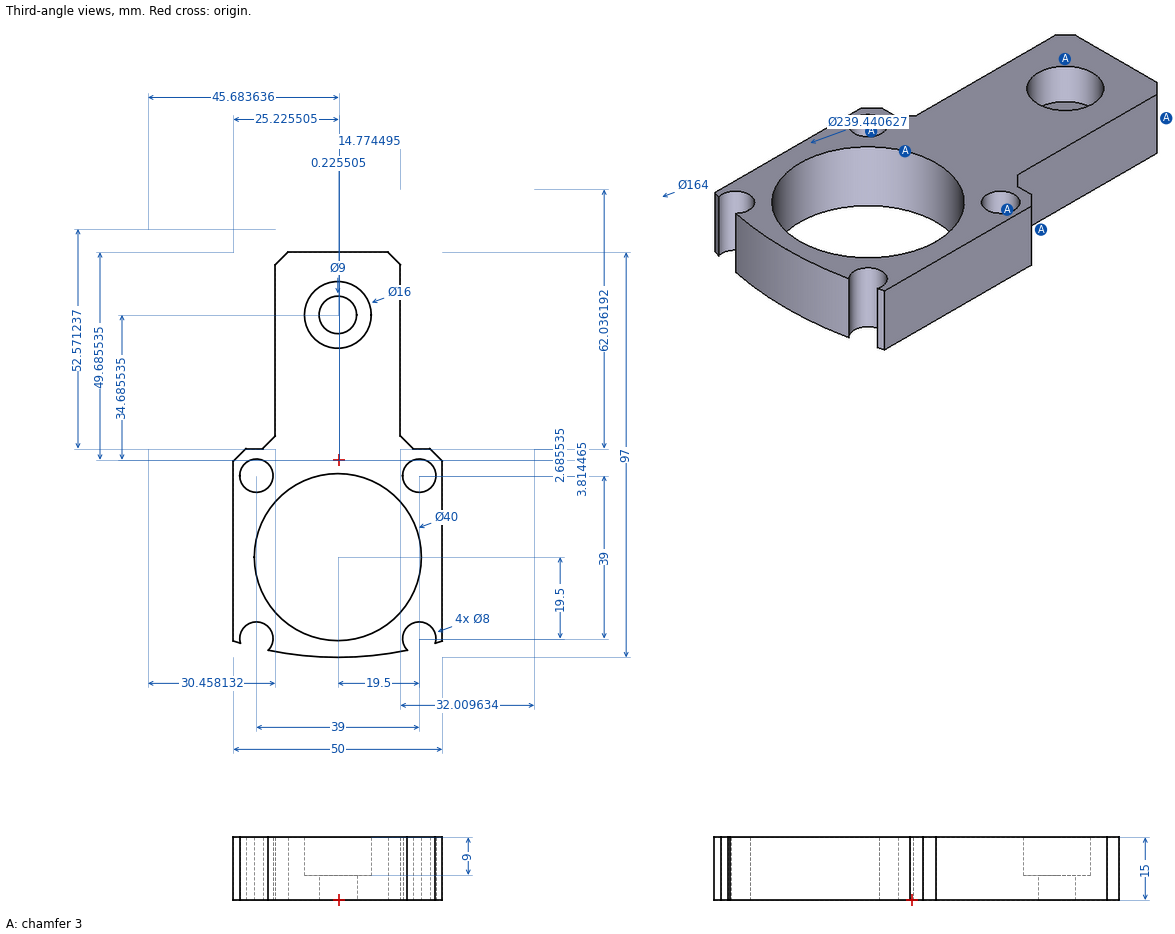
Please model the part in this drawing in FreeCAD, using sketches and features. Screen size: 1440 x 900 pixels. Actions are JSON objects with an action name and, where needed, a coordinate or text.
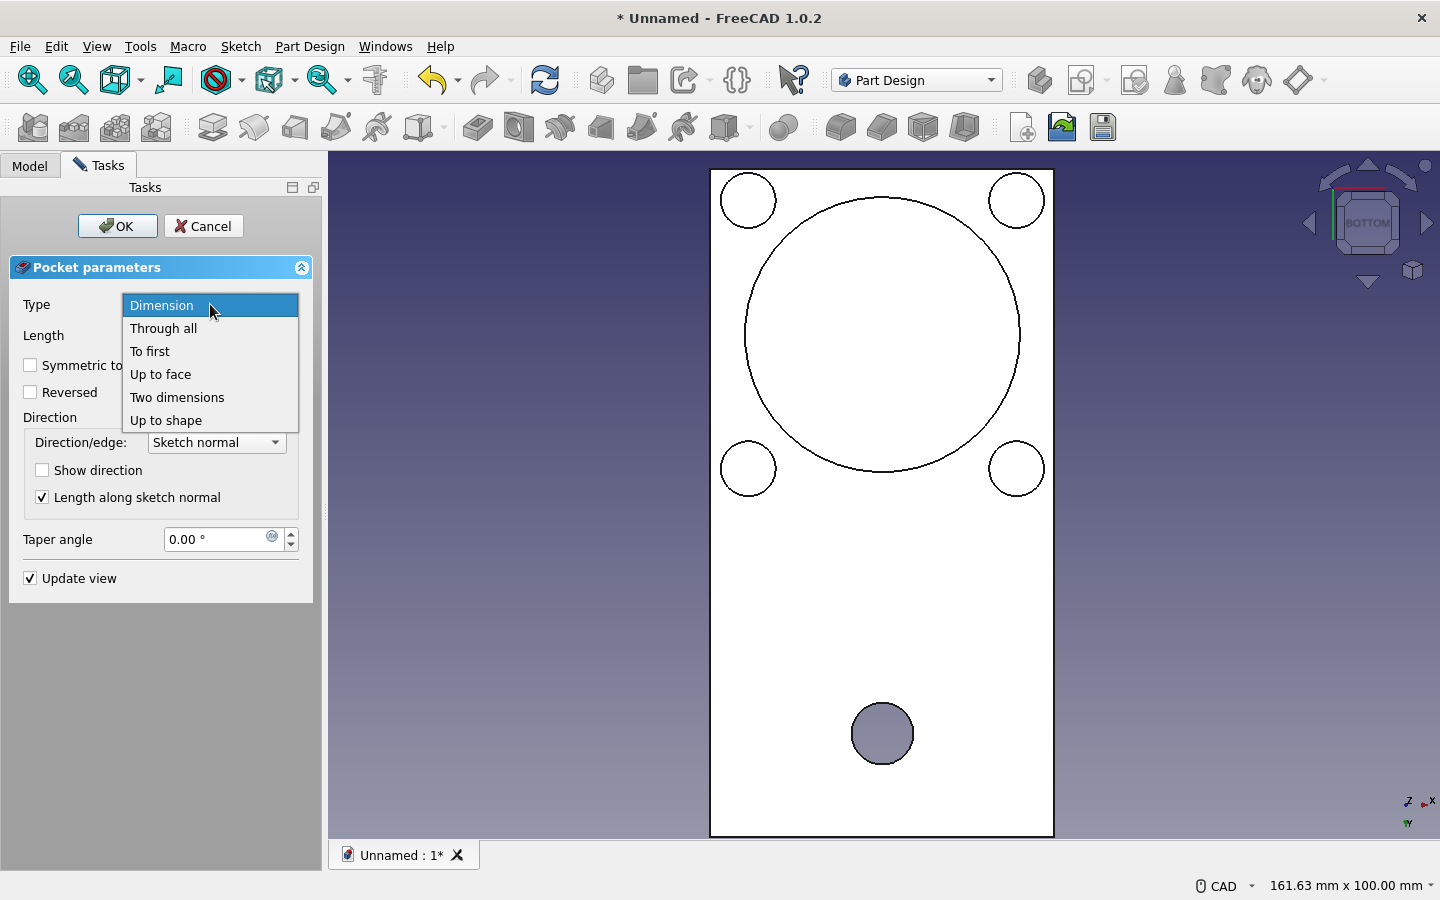
{"action": "left_click", "coordinate": [208, 328]}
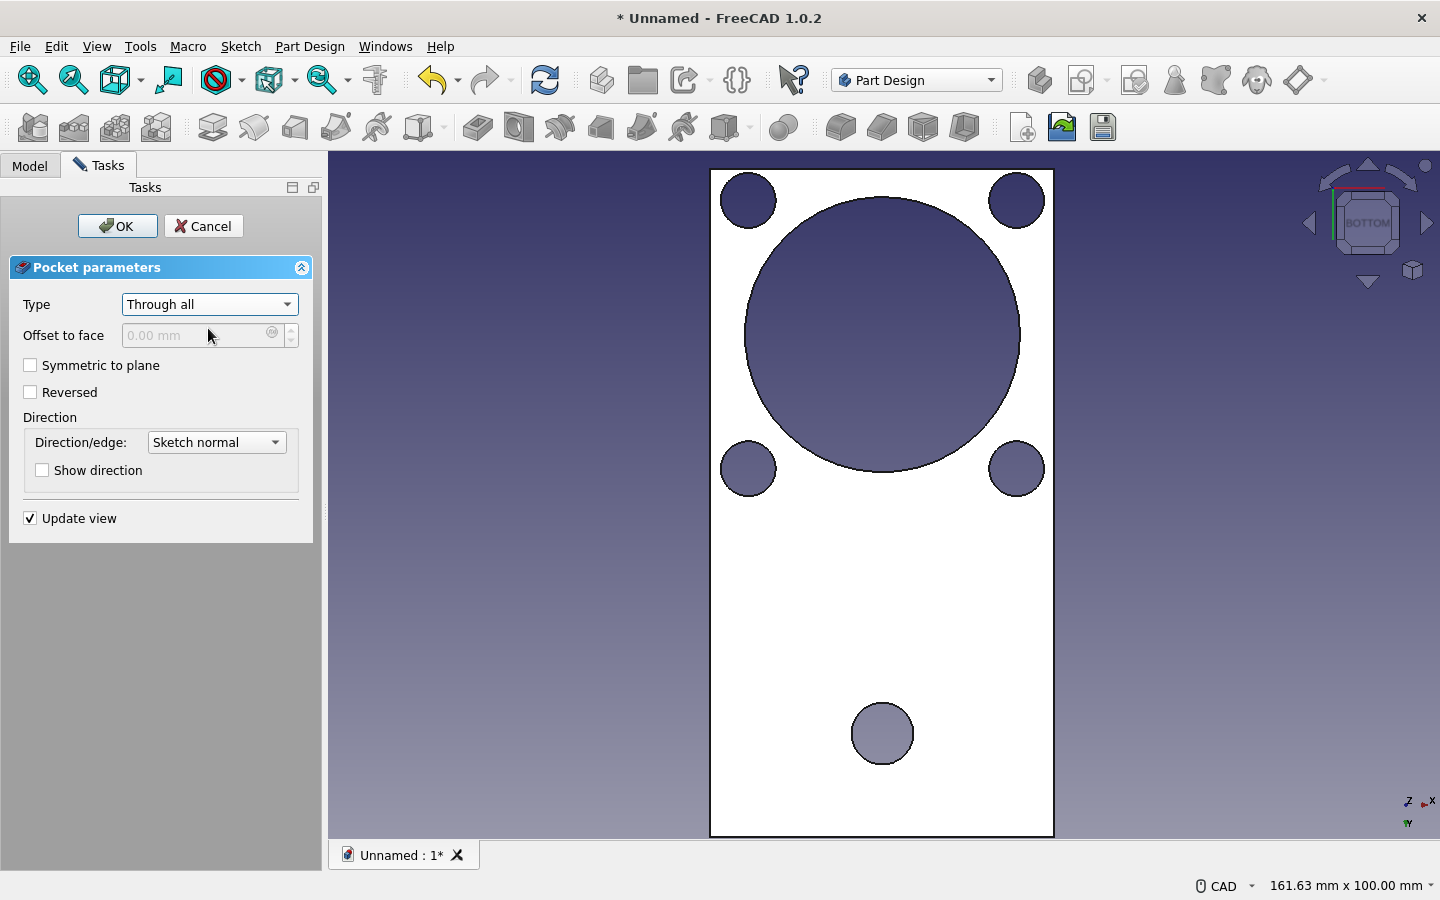
{"action": "left_click", "coordinate": [118, 226]}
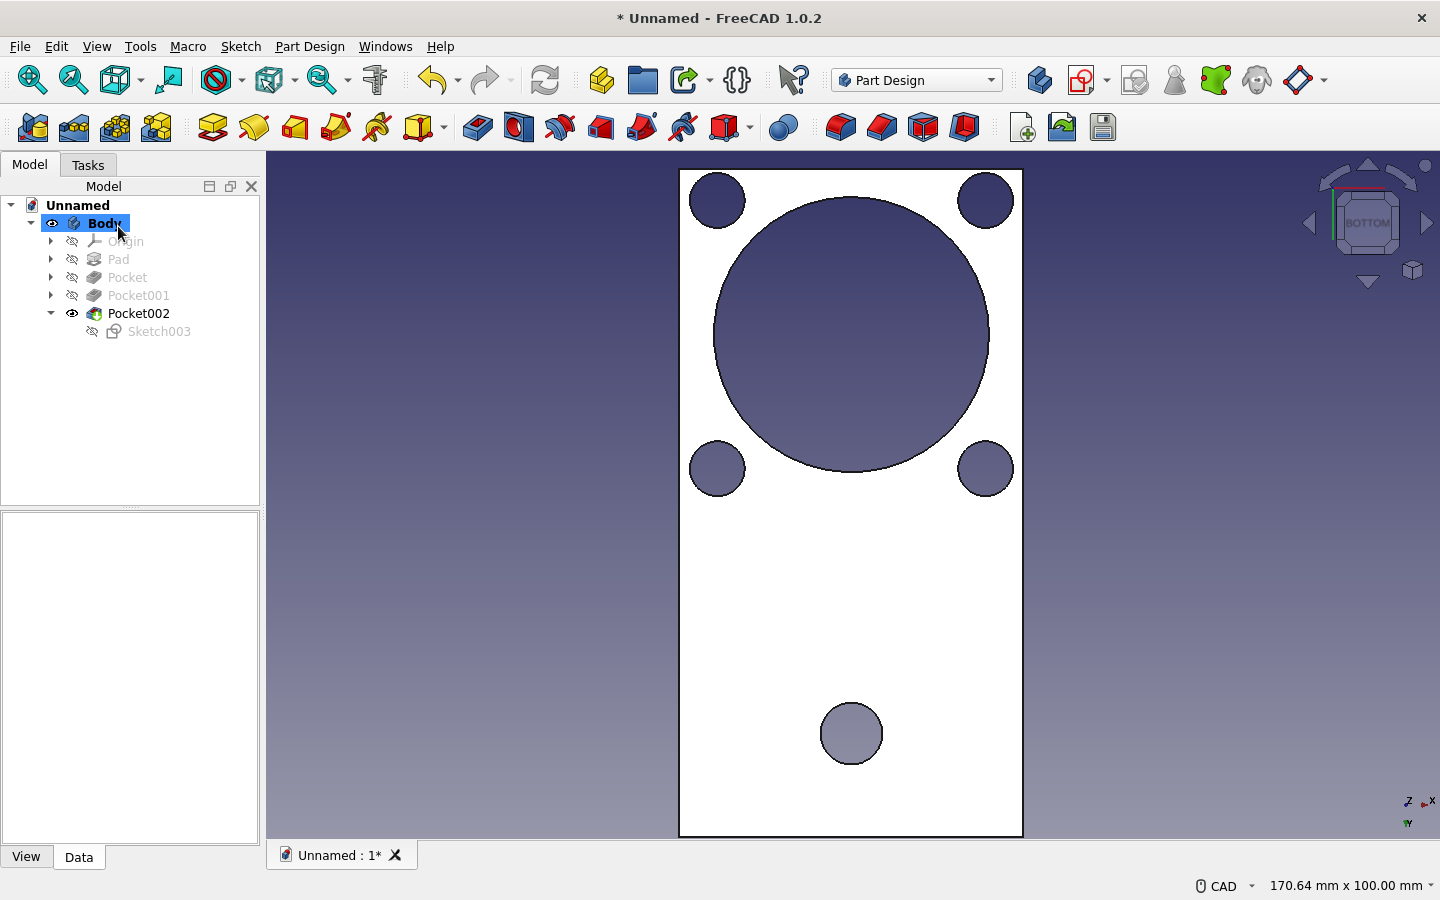
{"action": "key", "text": "0"}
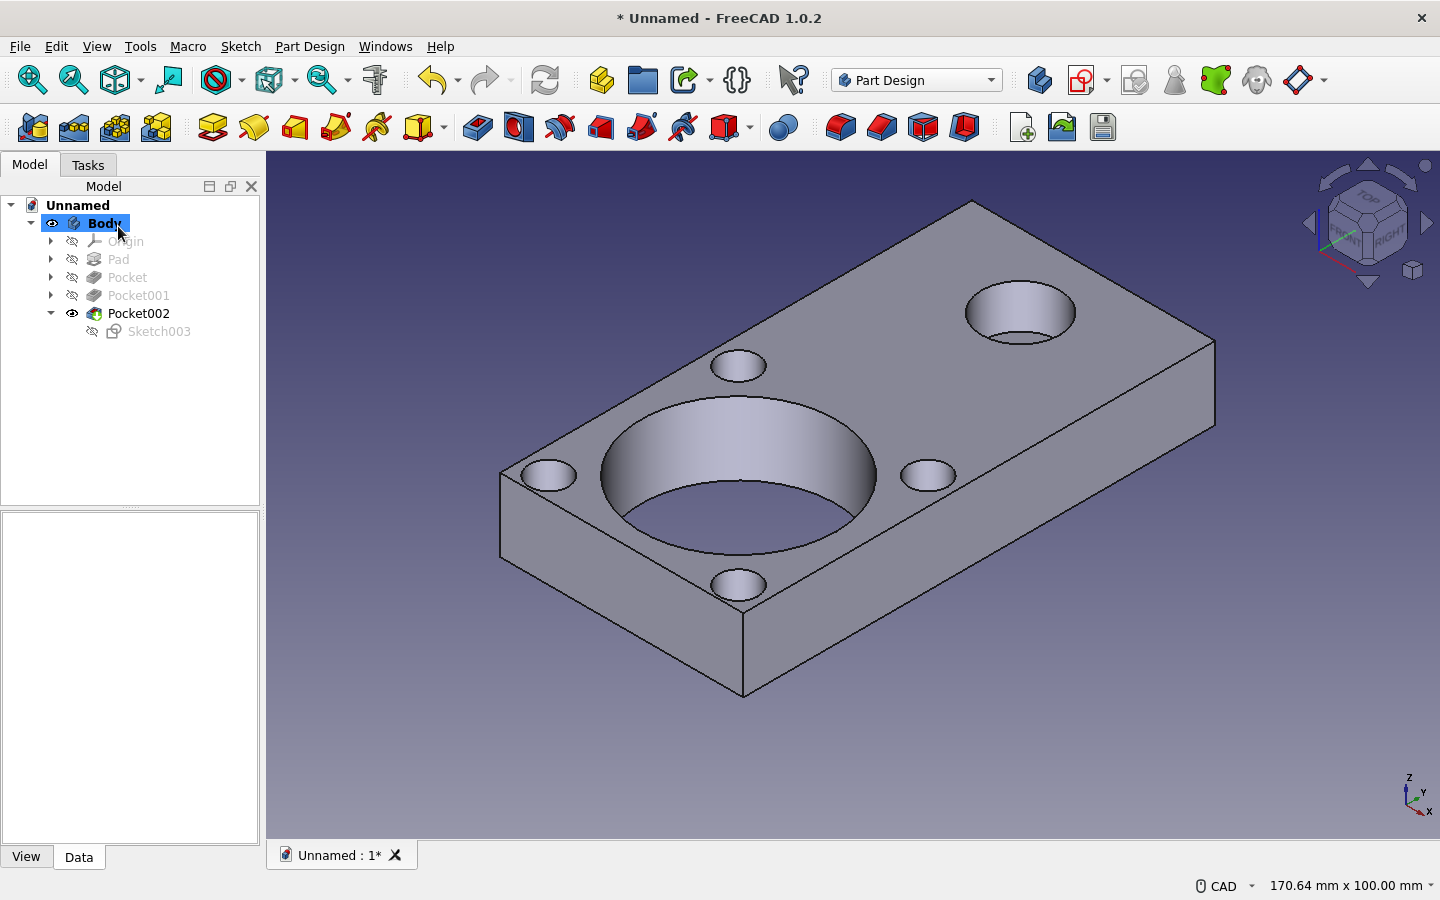
{"action": "left_click", "coordinate": [960, 387]}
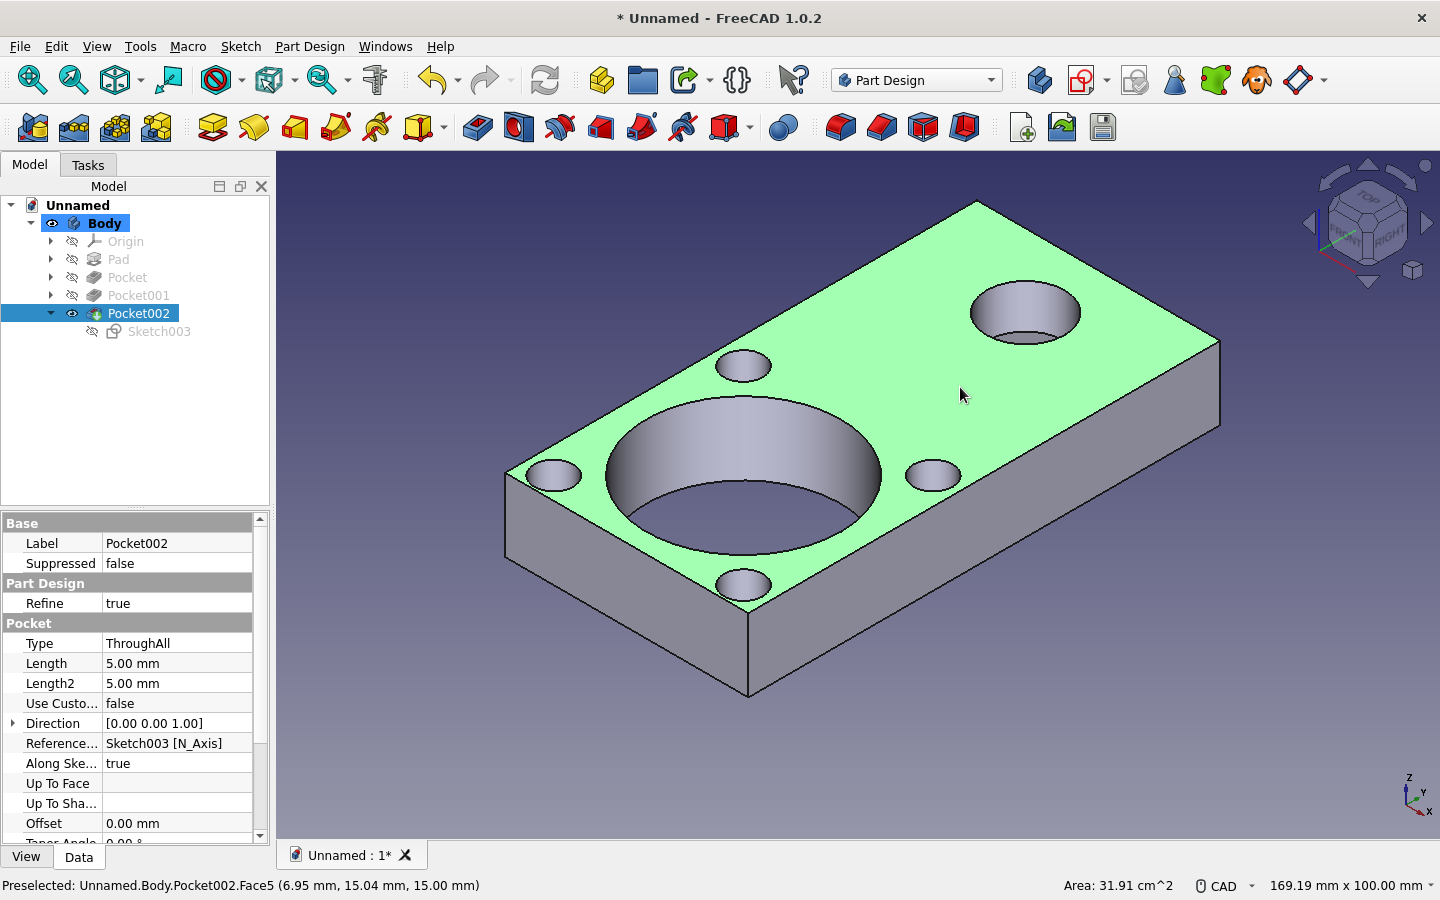
{"action": "left_click", "coordinate": [1080, 80]}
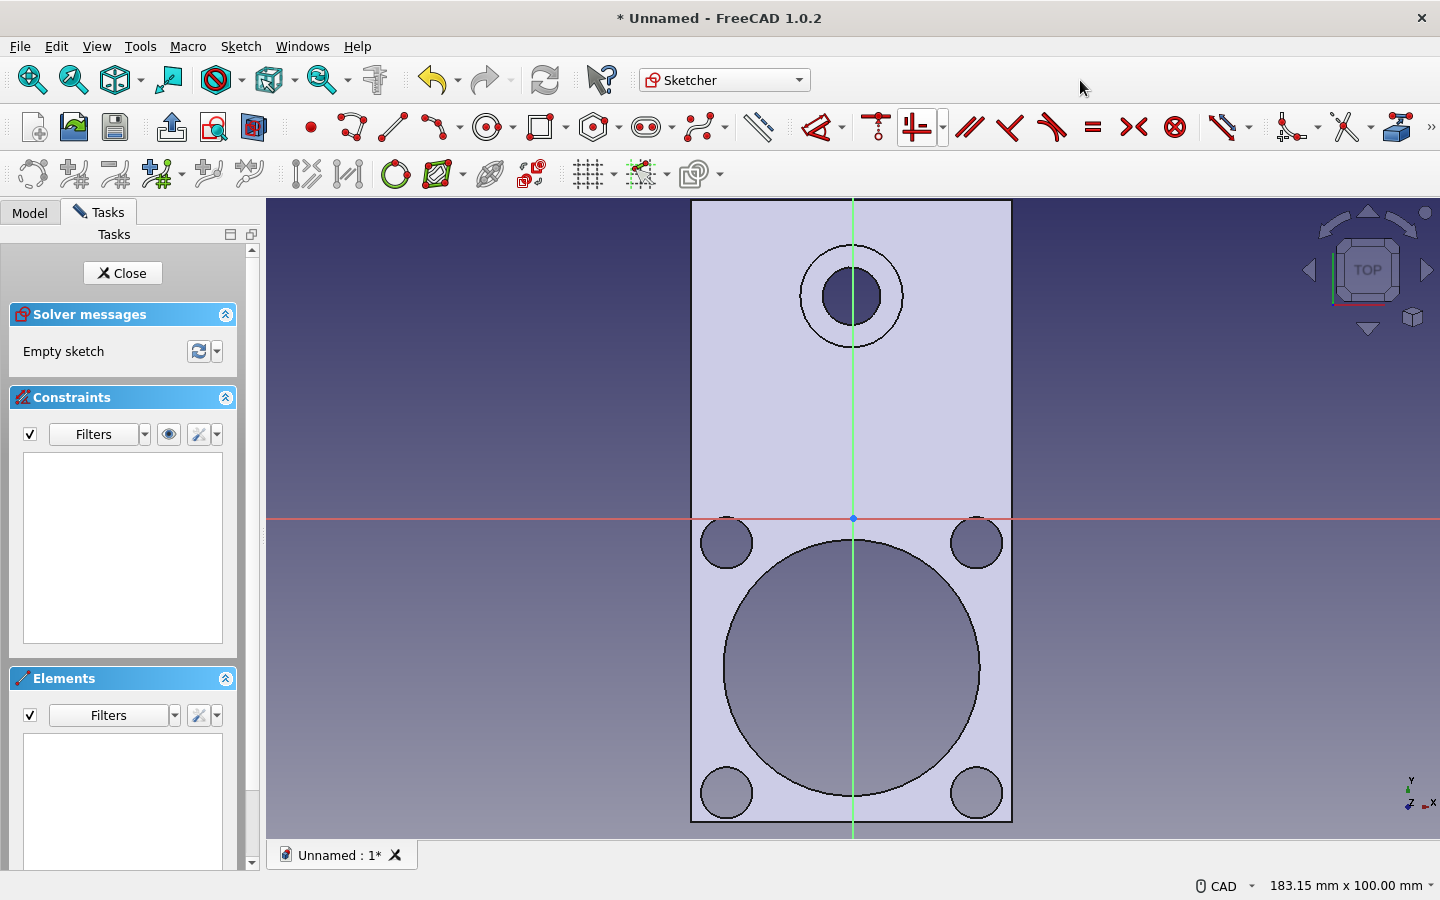
{"action": "scroll", "coordinate": [638, 811], "scroll_direction": "down", "scroll_amount": 2}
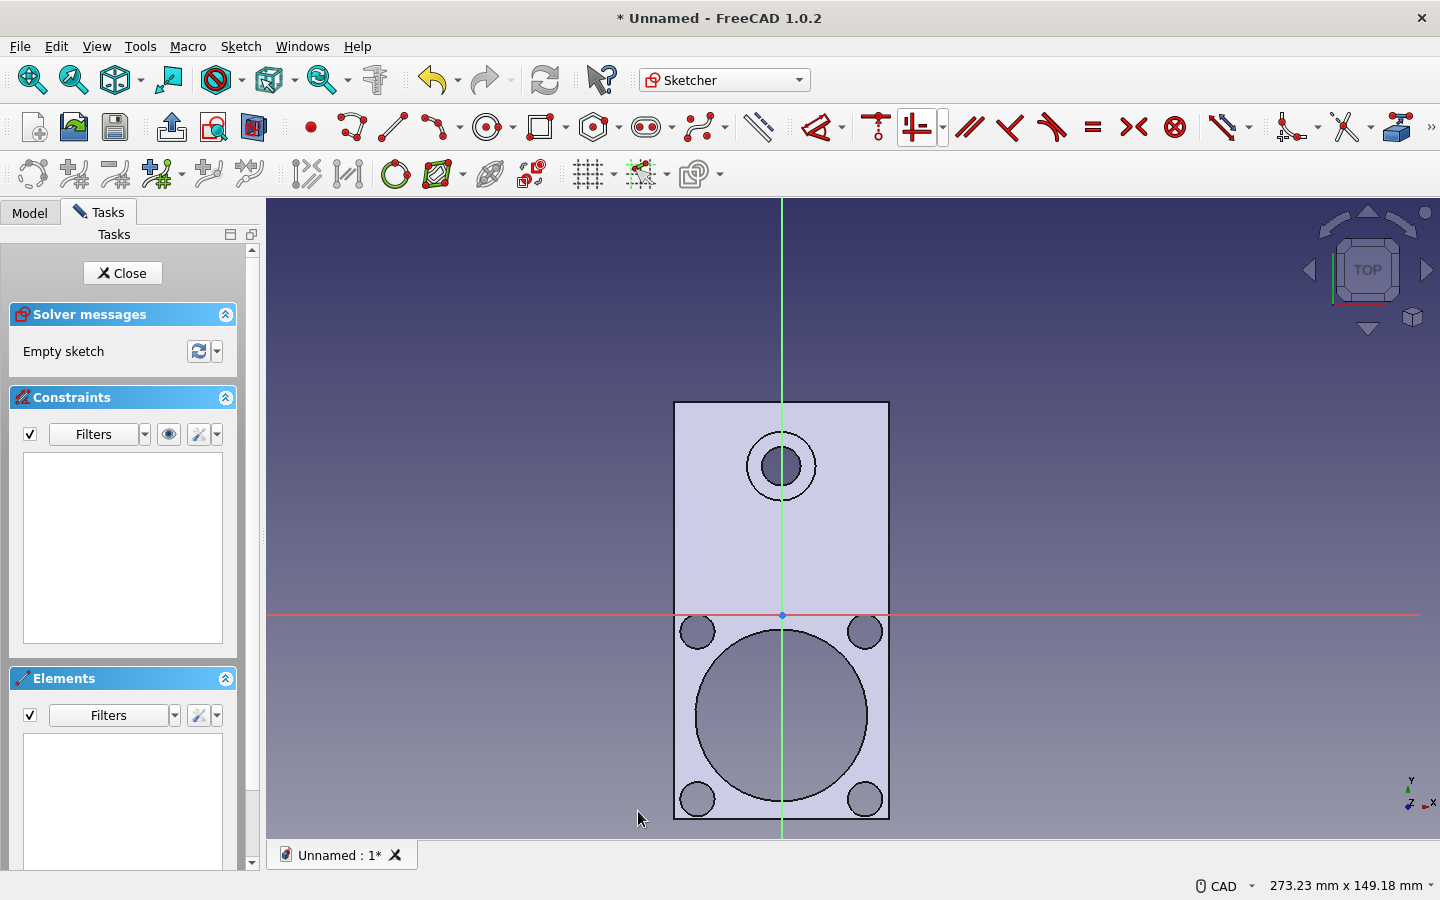
{"action": "scroll", "coordinate": [785, 390], "scroll_direction": "up", "scroll_amount": 2}